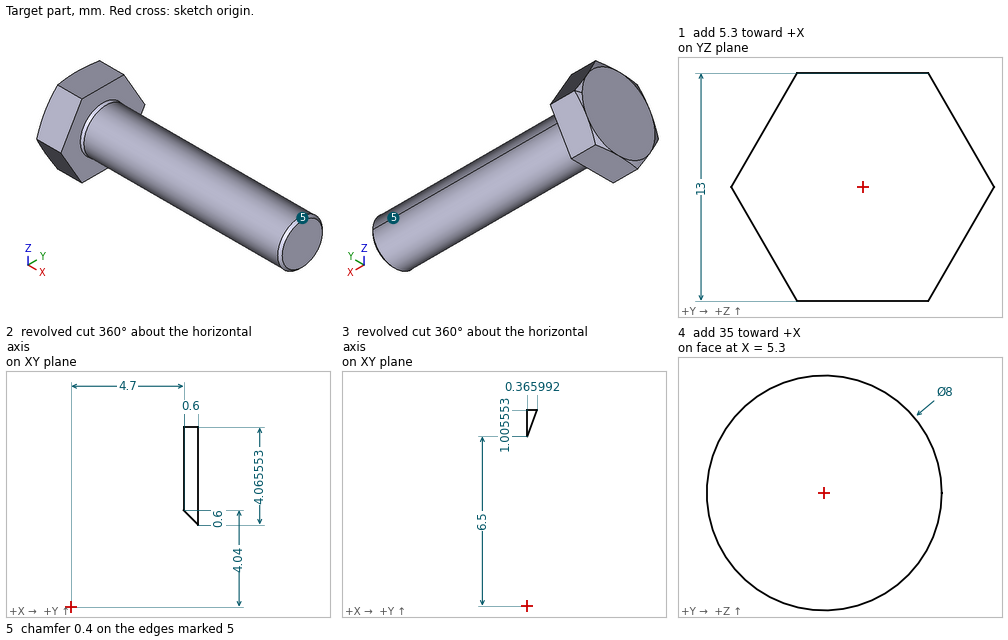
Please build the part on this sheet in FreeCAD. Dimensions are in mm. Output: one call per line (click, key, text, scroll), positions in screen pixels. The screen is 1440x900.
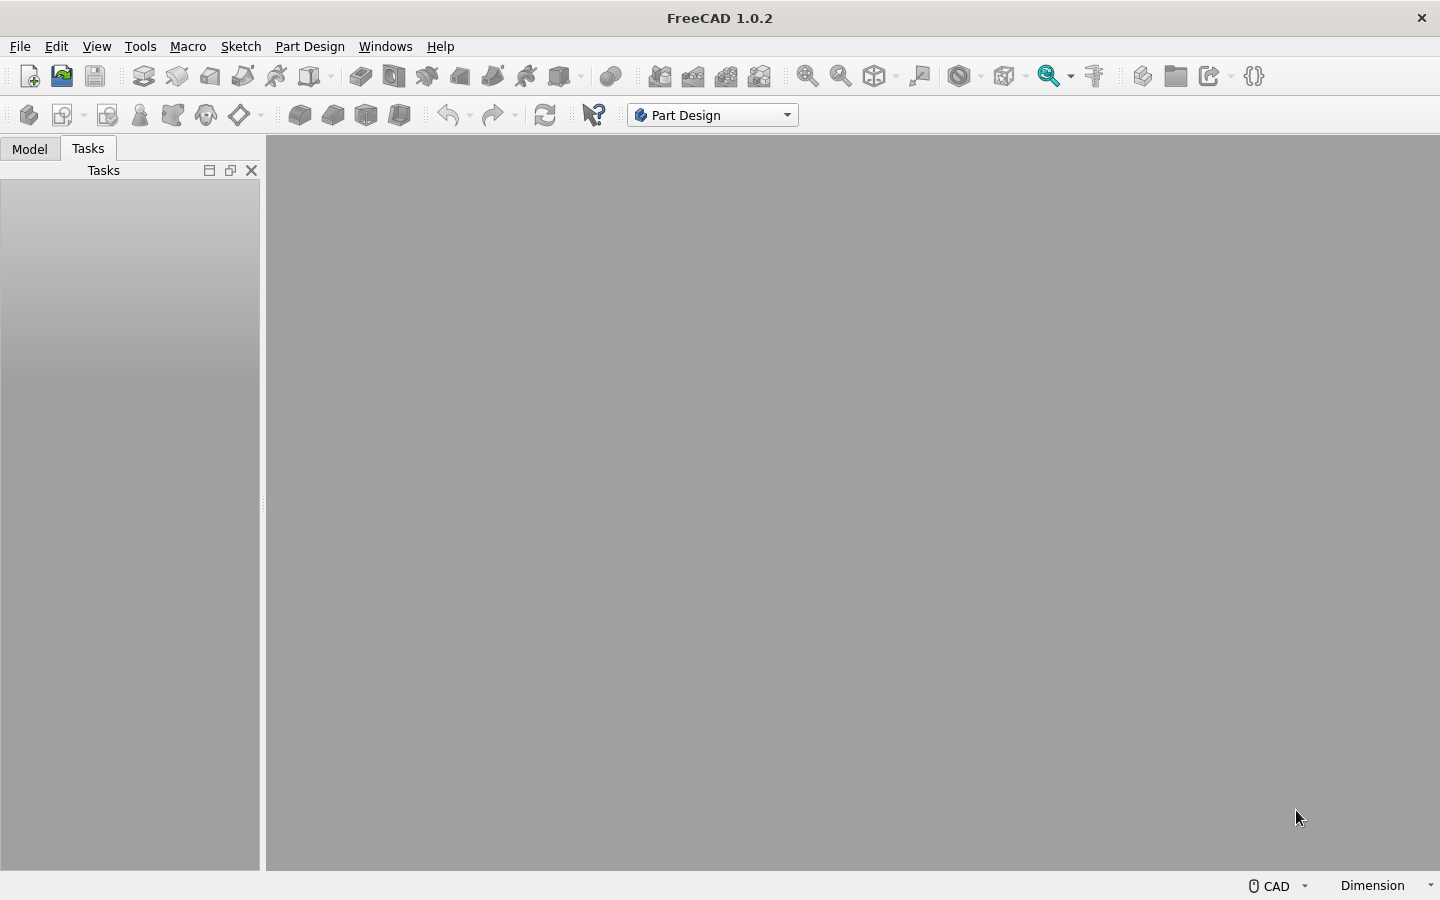
key(ctrl+n)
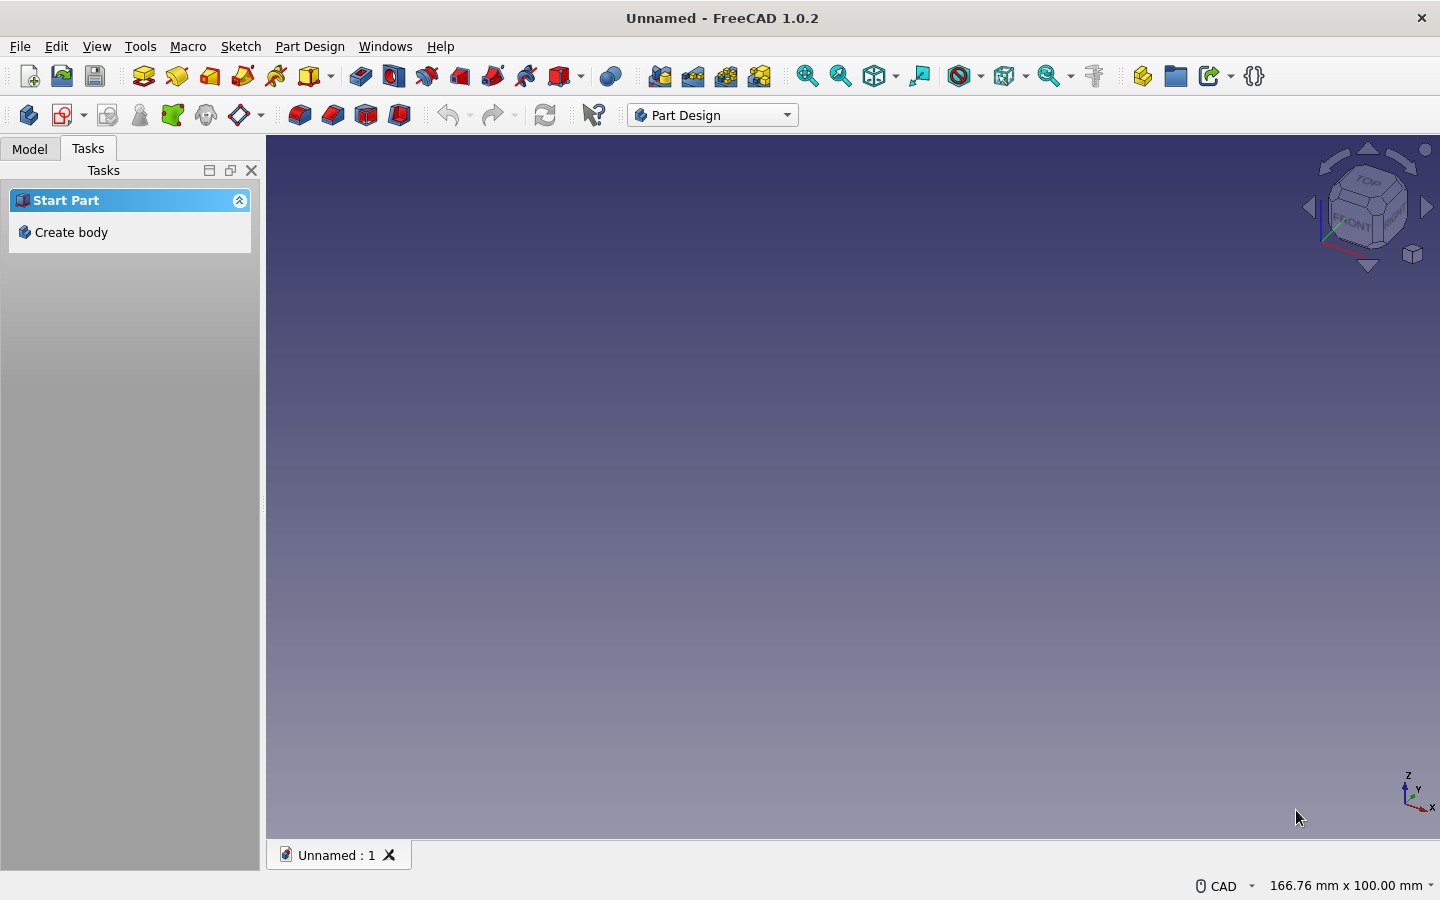
click(62, 116)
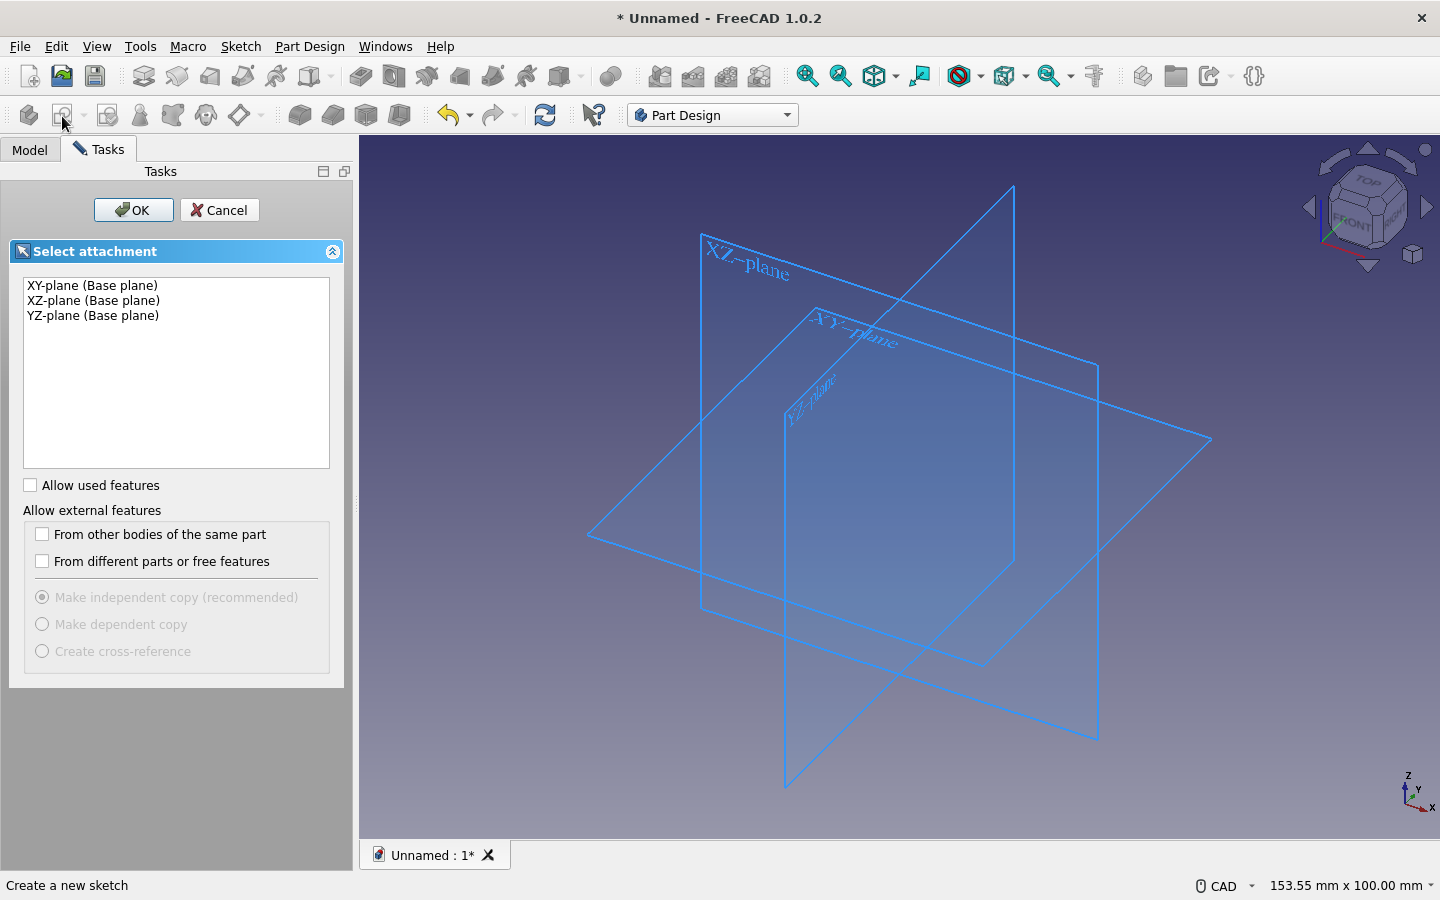
click(84, 316)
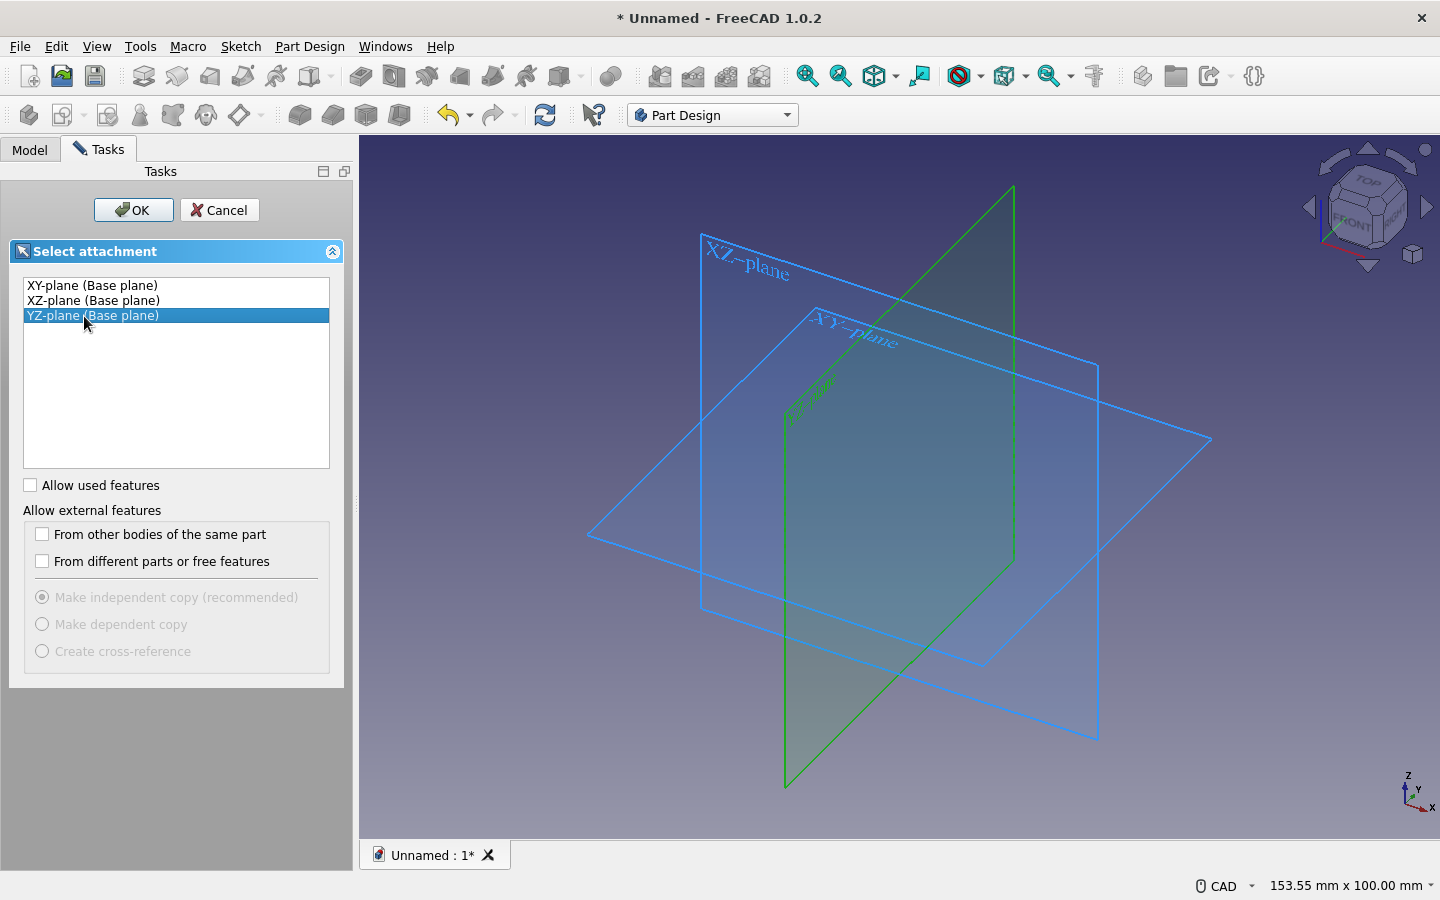
click(134, 210)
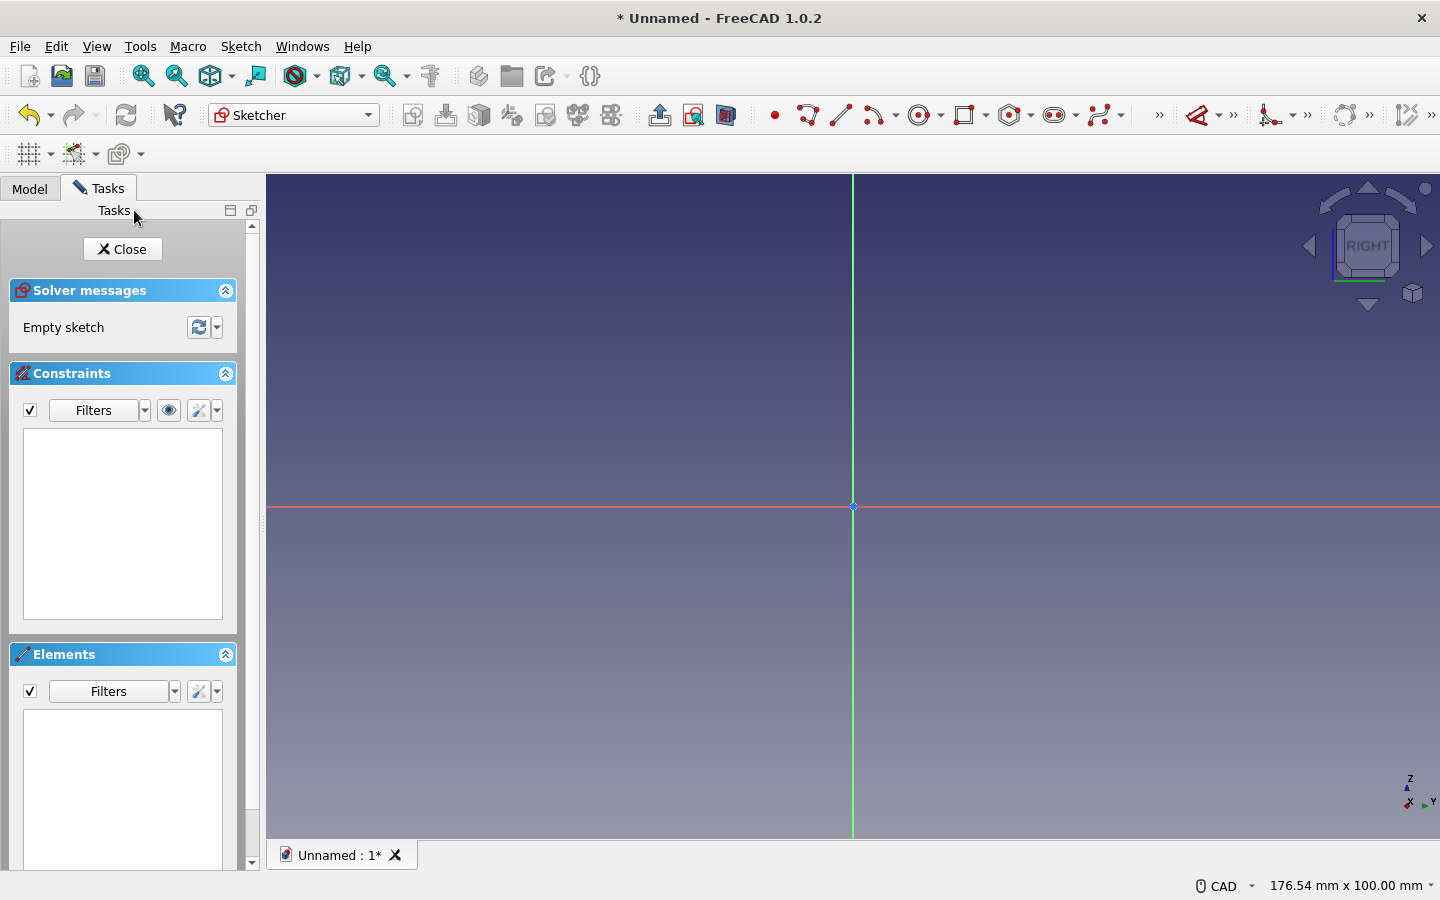
scroll(870, 506, up, 8)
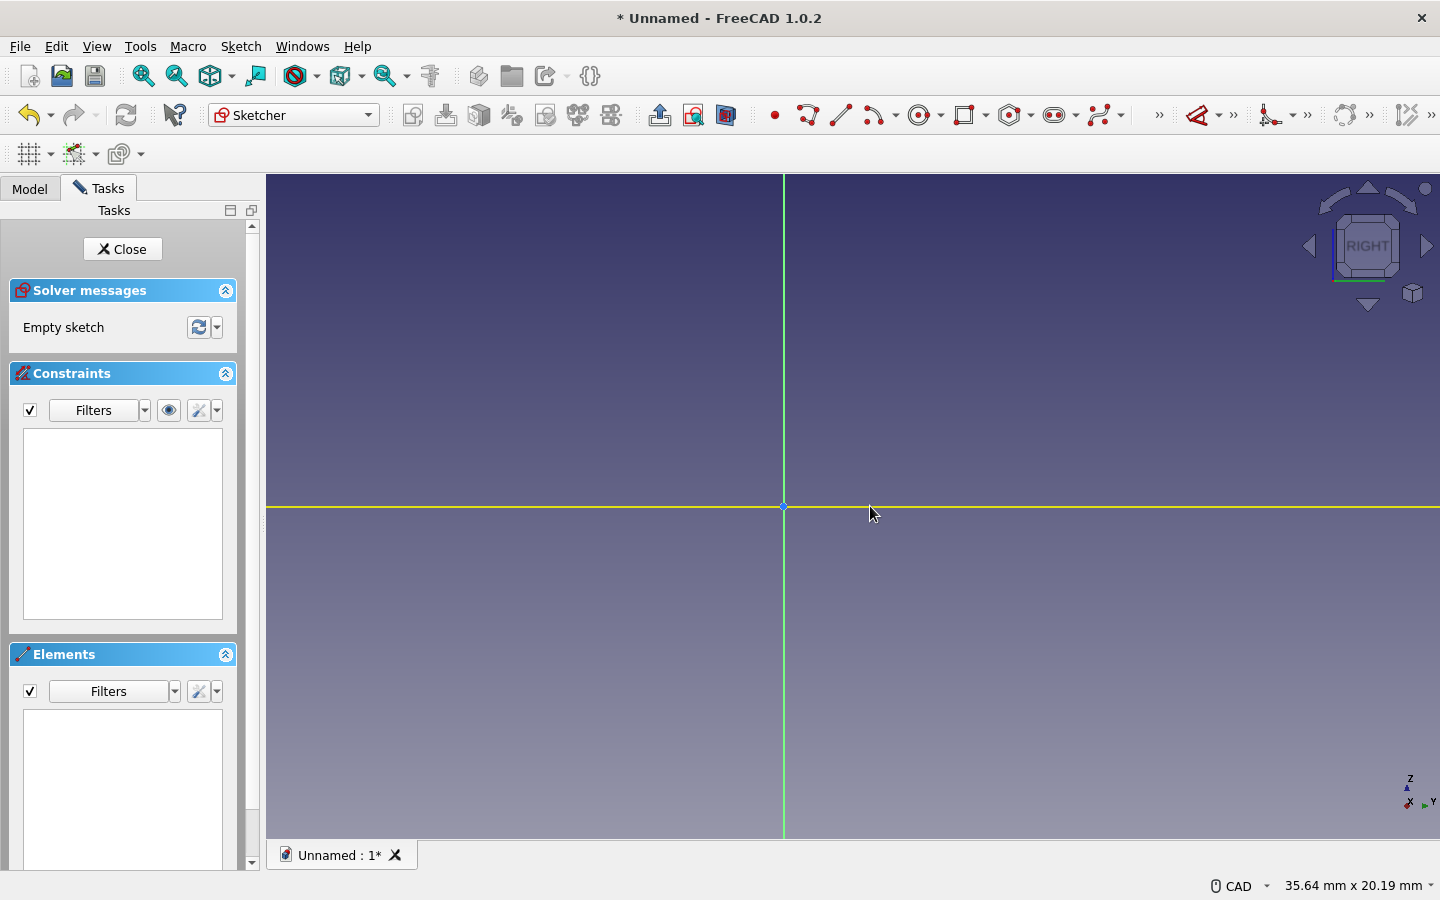
key(g)
key(p)
key(6)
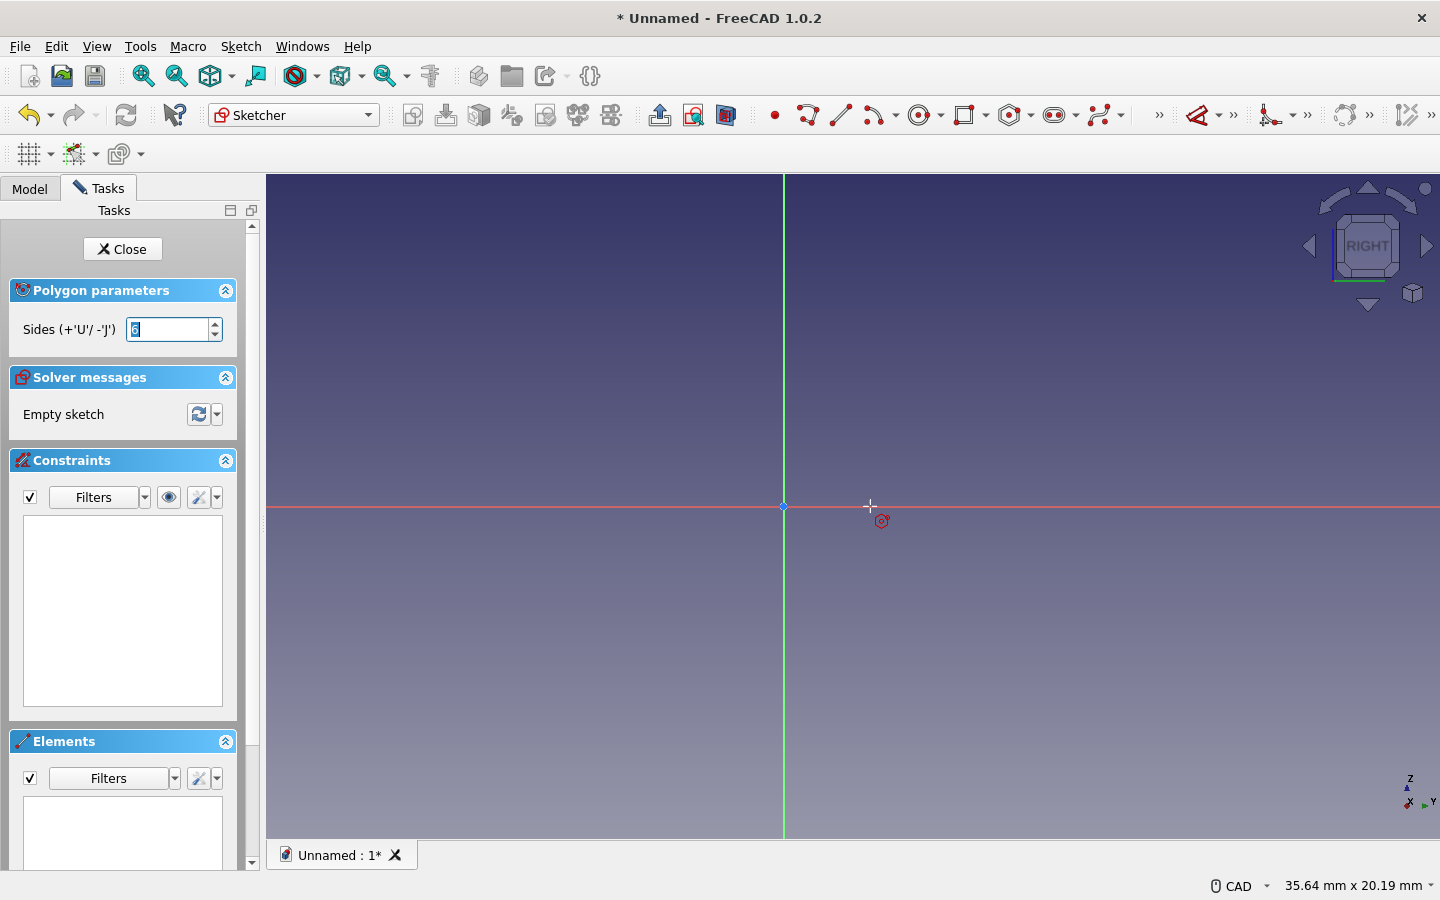
click(784, 506)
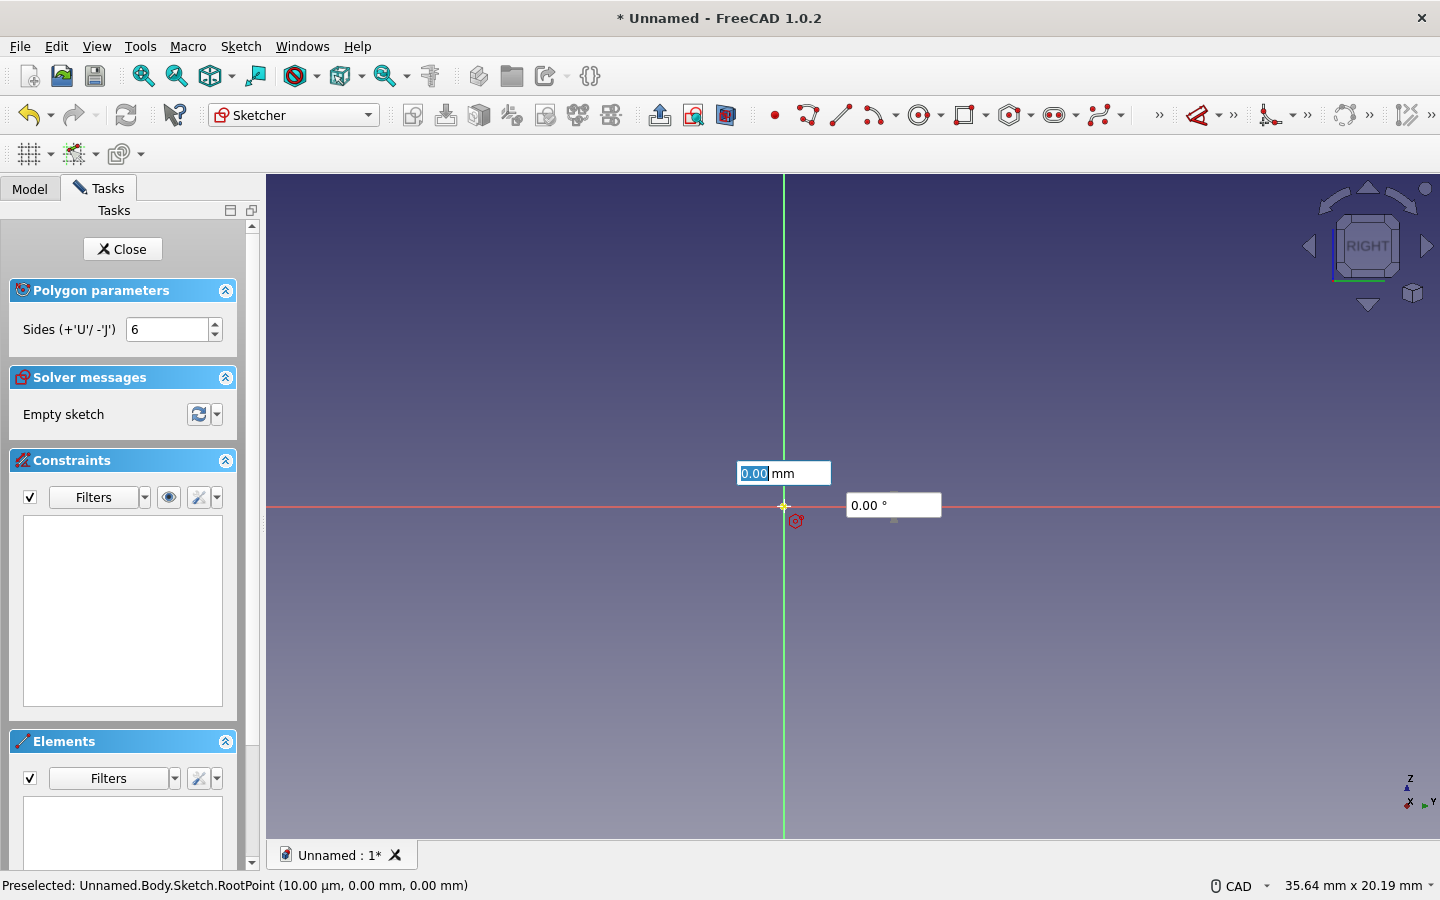
click(1031, 506)
right_click(1031, 506)